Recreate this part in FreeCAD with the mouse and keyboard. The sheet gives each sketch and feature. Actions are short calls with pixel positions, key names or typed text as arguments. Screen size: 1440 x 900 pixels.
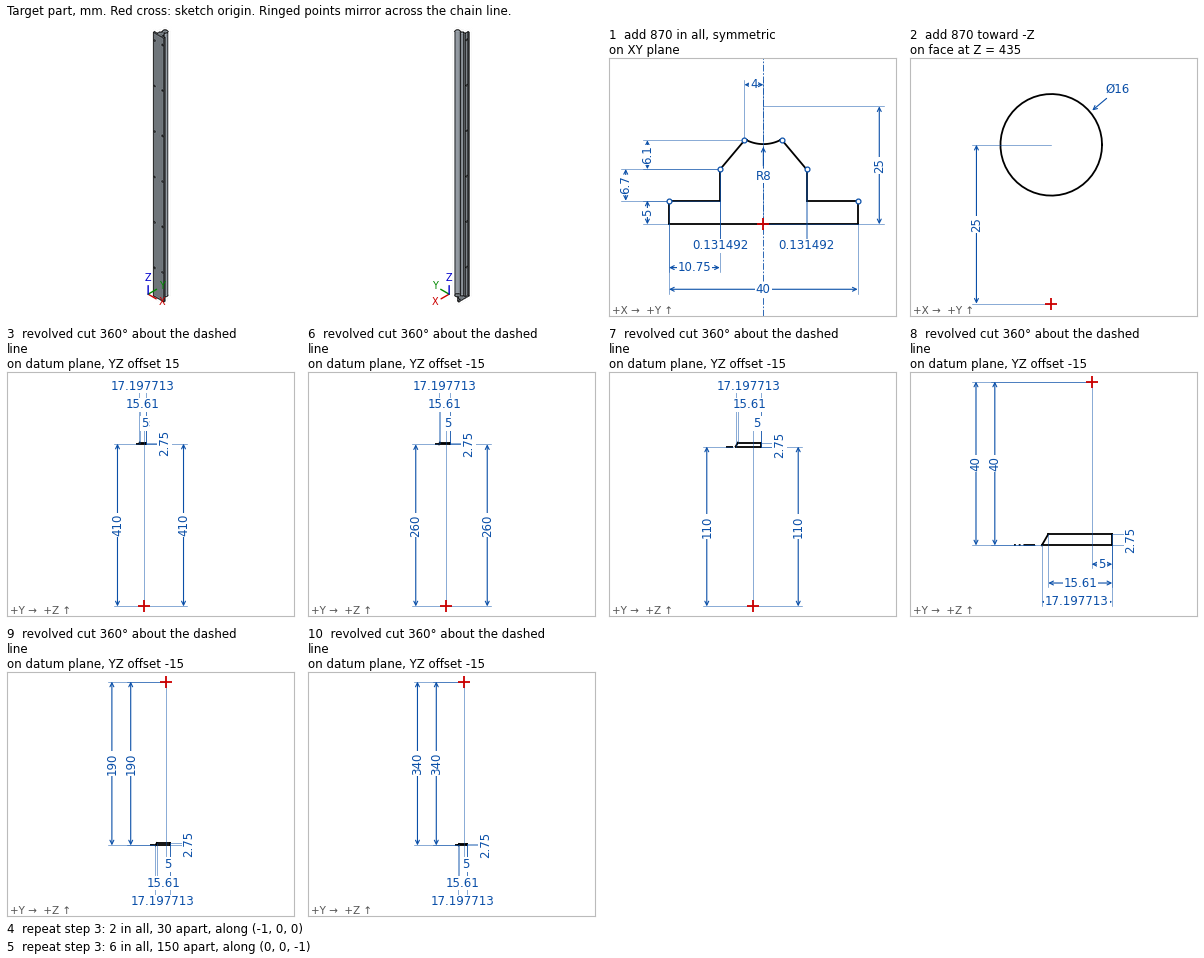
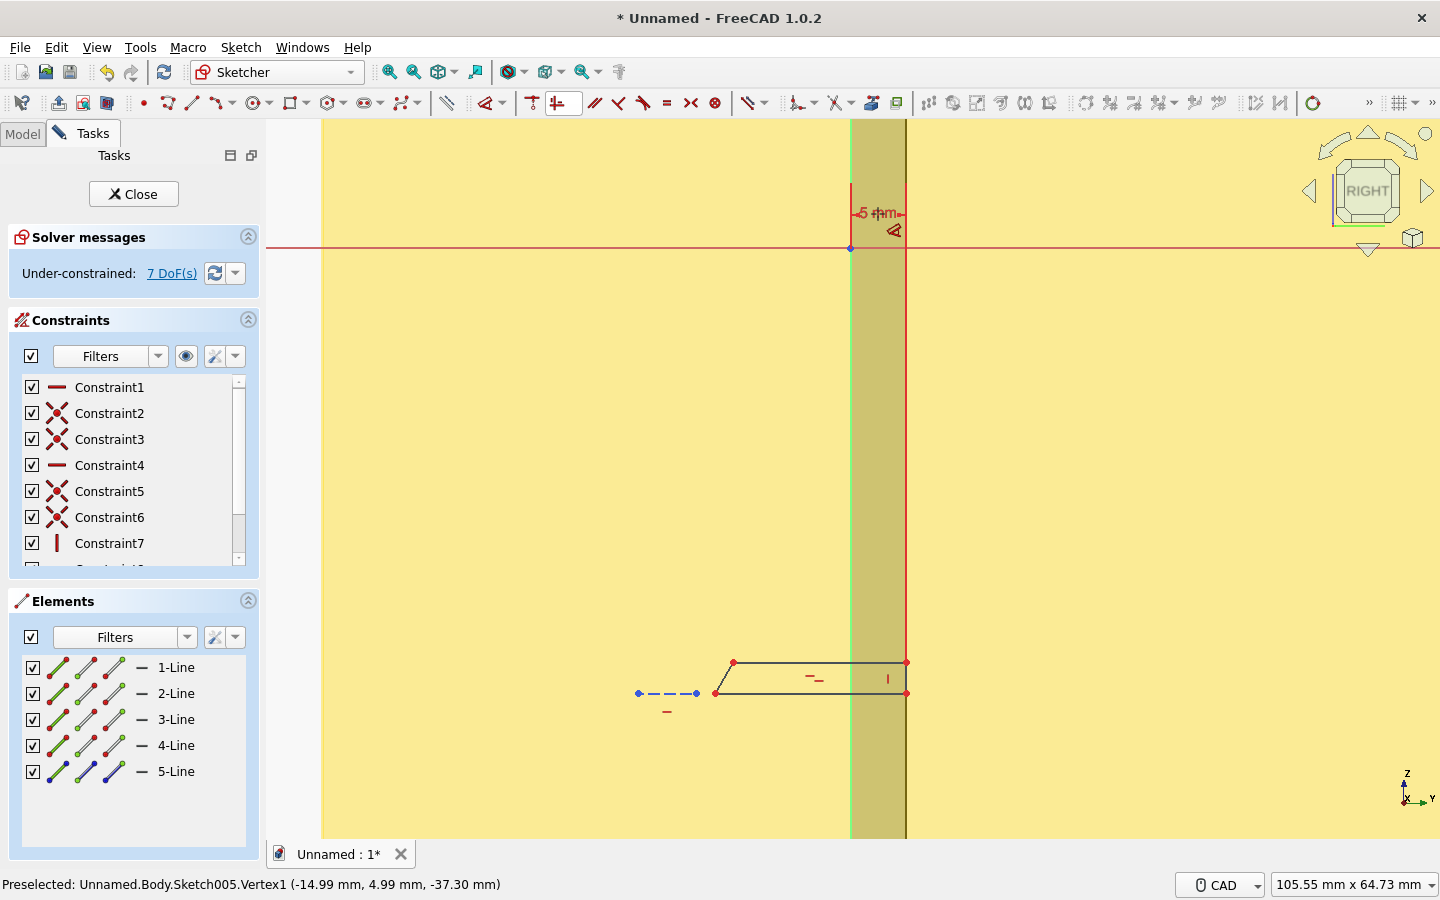
click(715, 694)
click(885, 471)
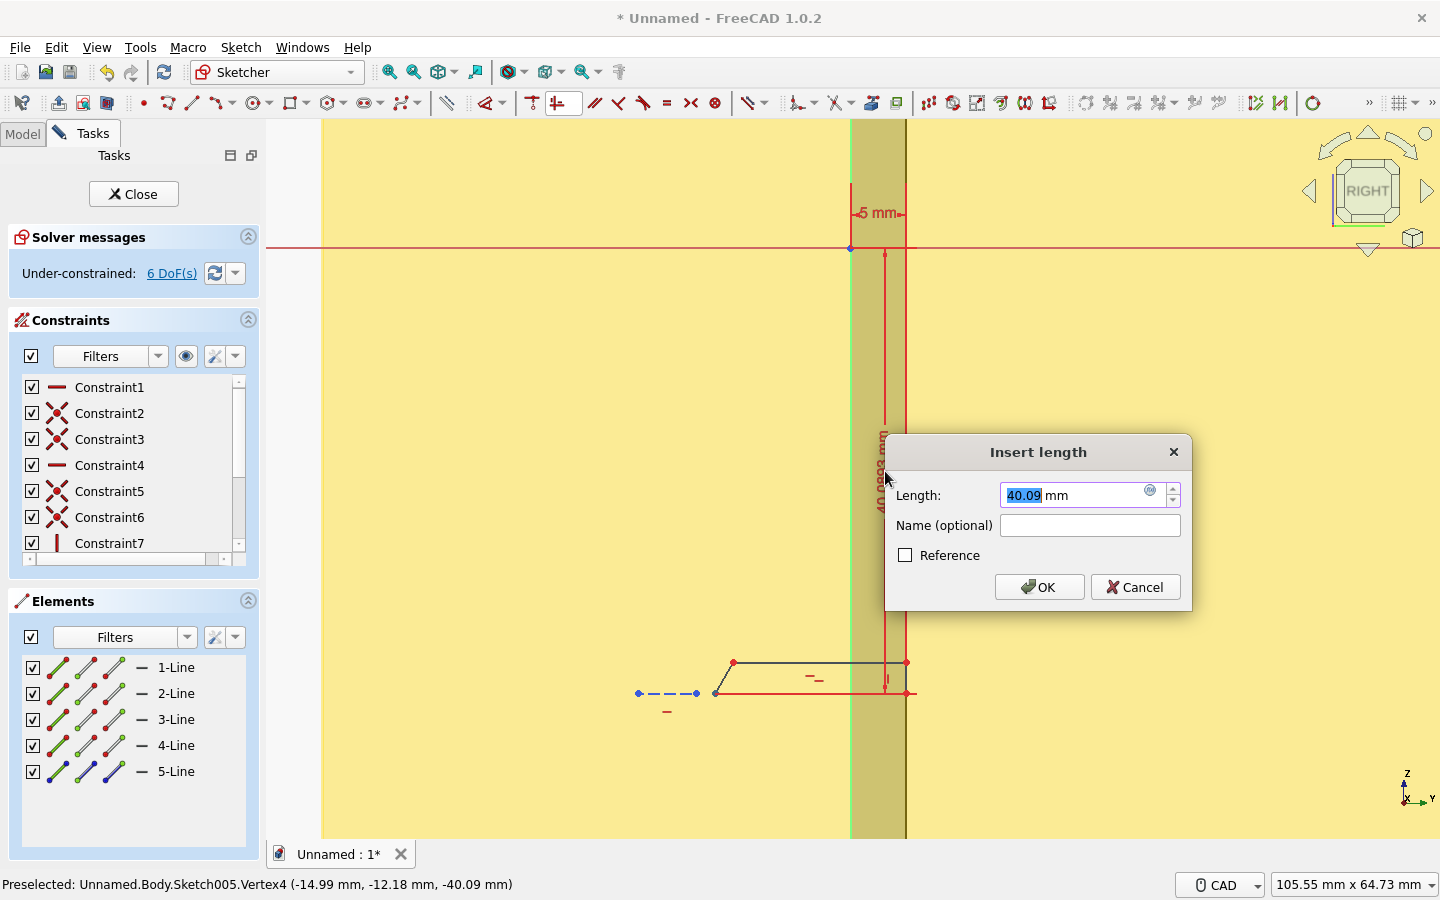
text(40)
key(Return)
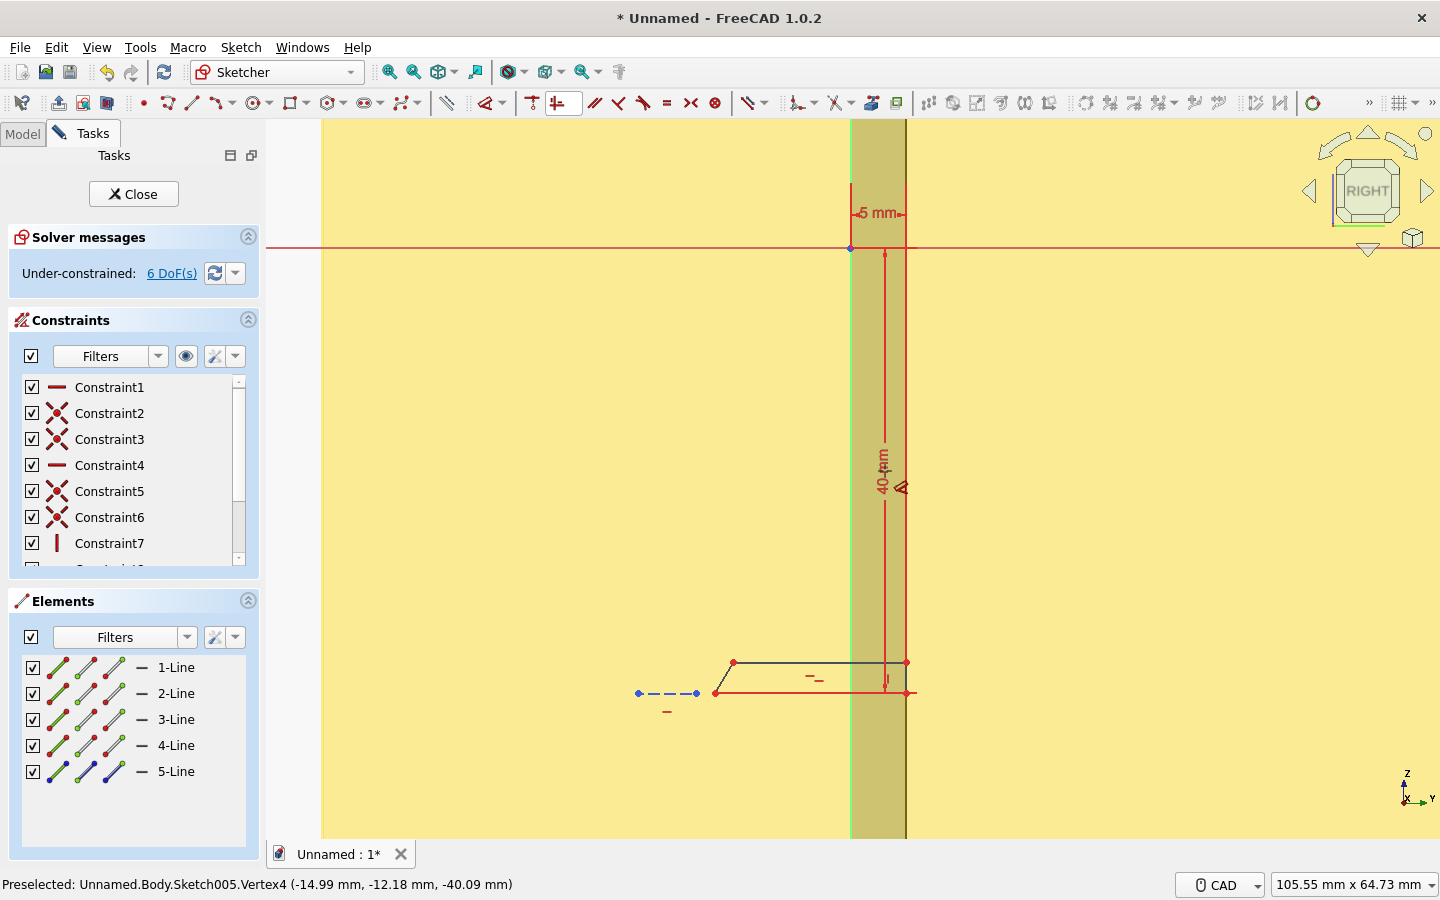
click(696, 694)
click(885, 368)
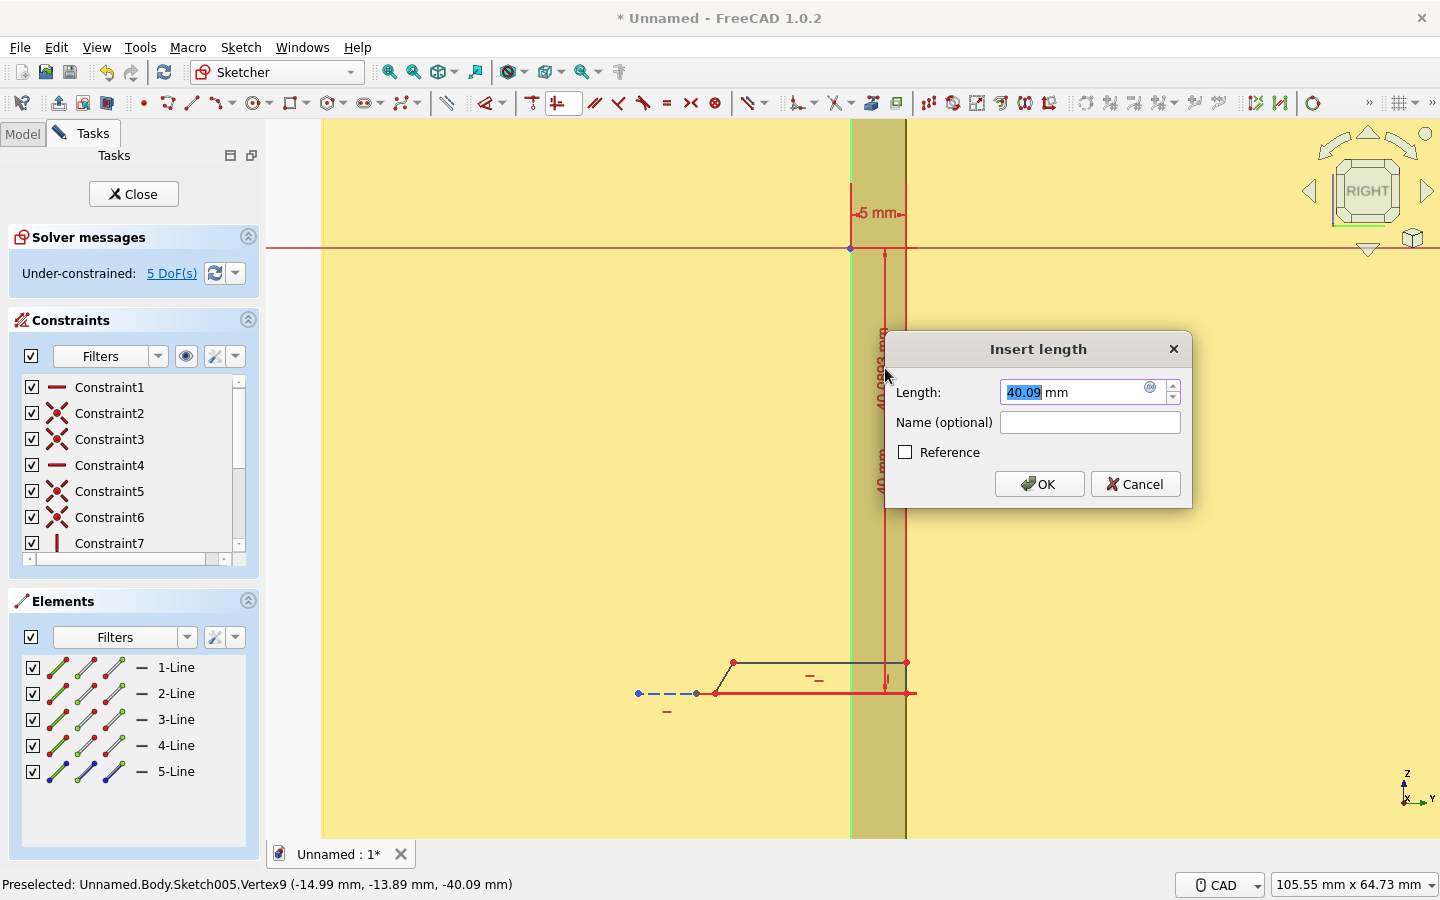
text(40)
key(Return)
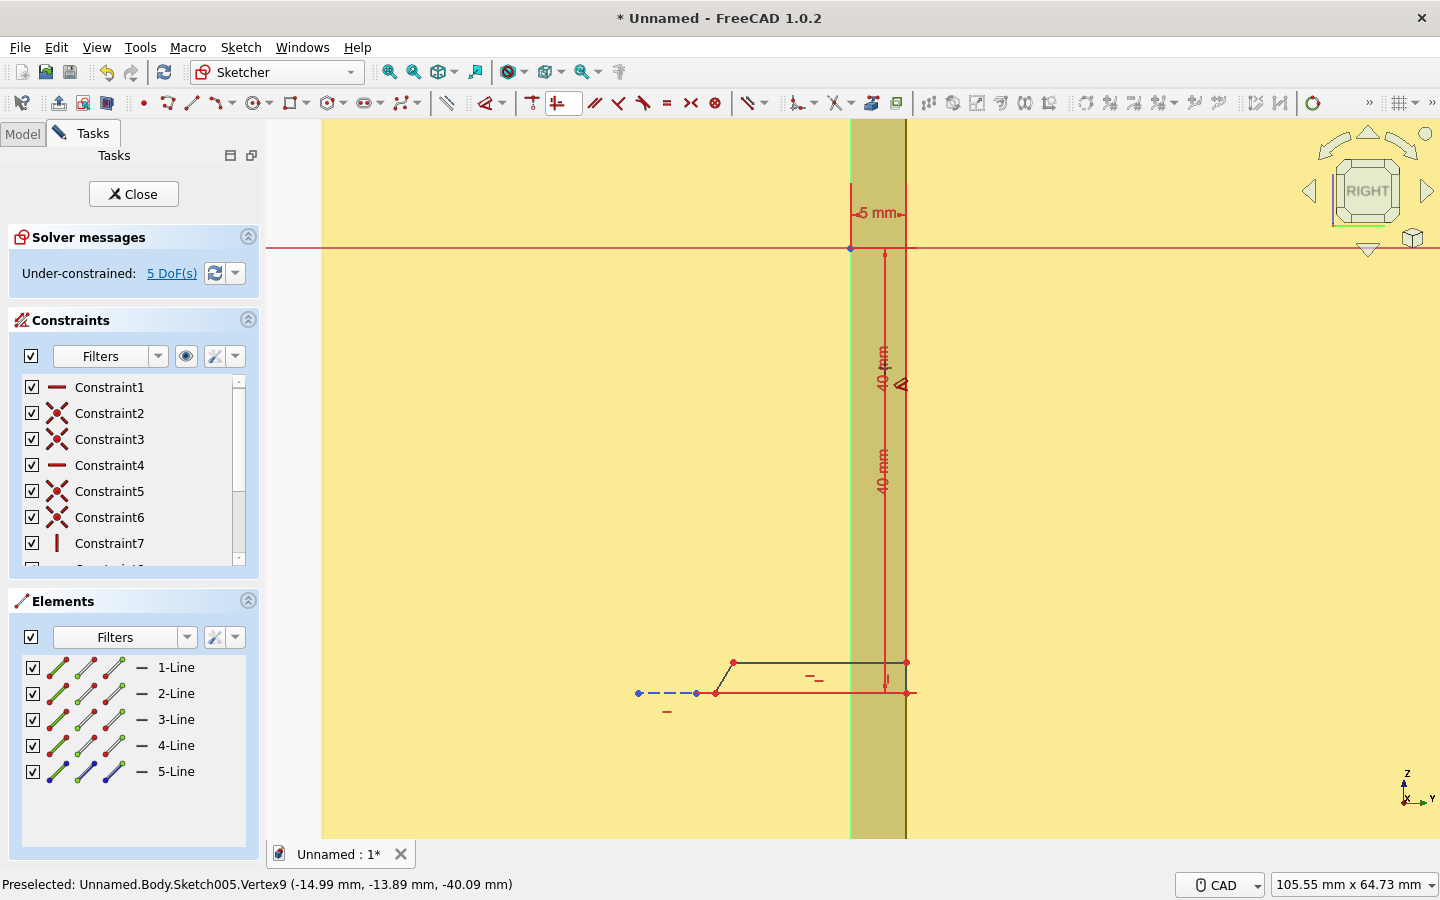
scroll(906, 684, up, 3)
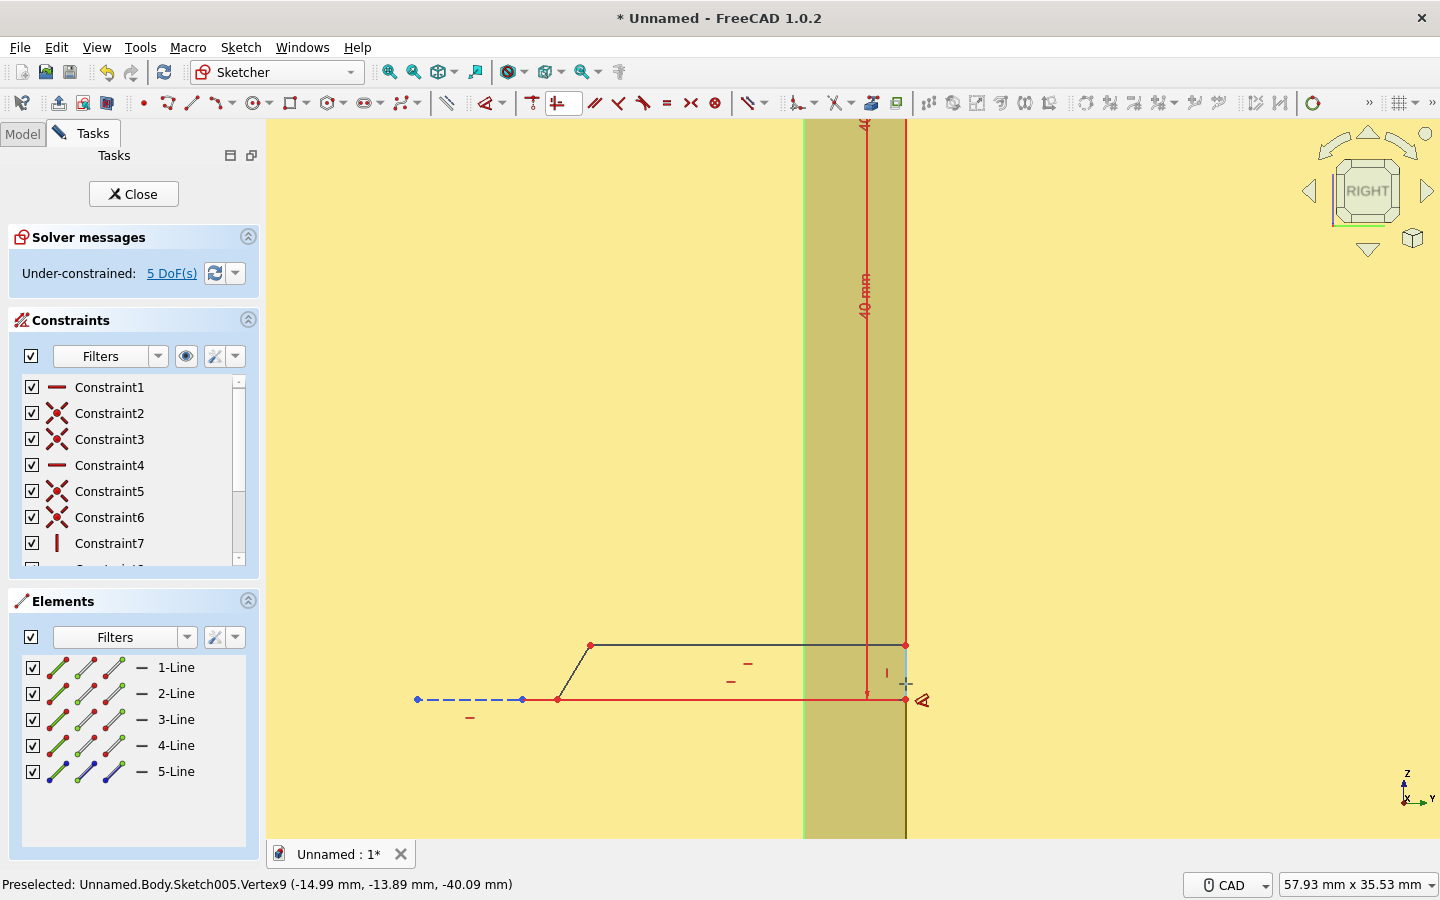
click(906, 683)
click(940, 672)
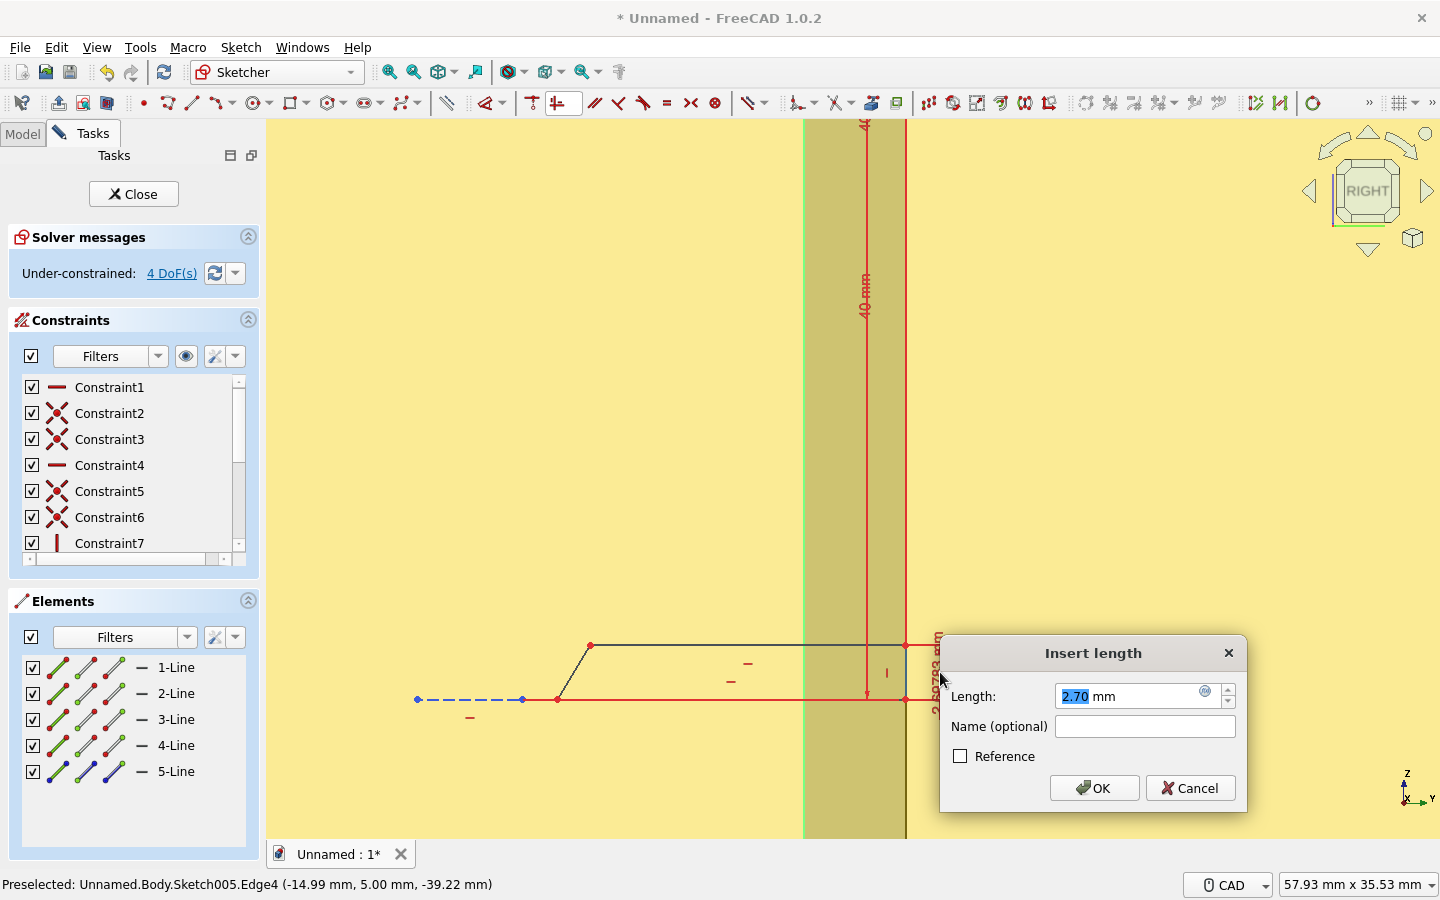
text(2.75)
key(Return)